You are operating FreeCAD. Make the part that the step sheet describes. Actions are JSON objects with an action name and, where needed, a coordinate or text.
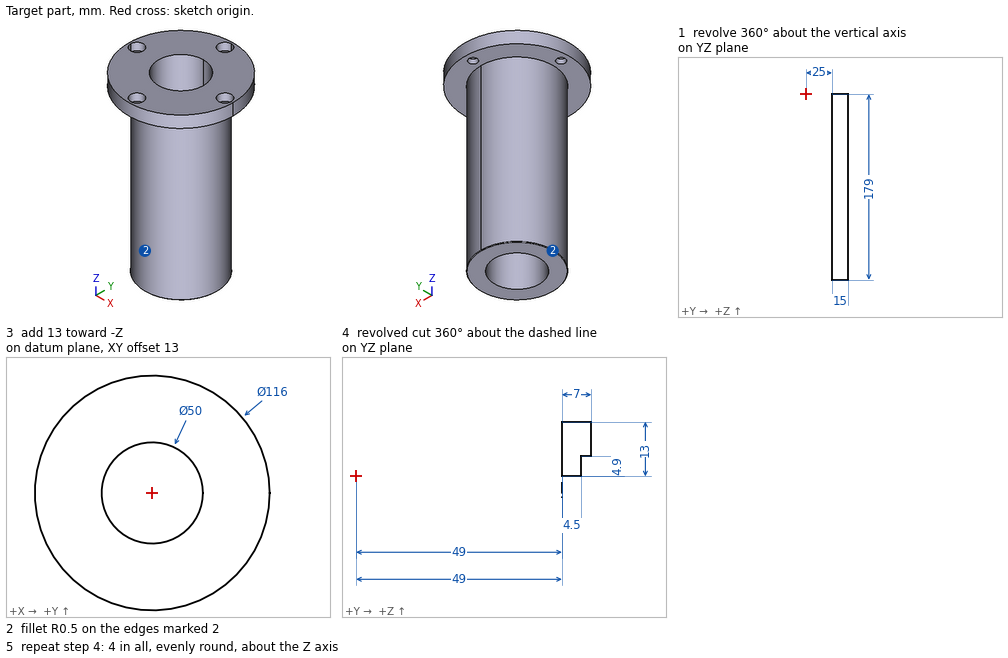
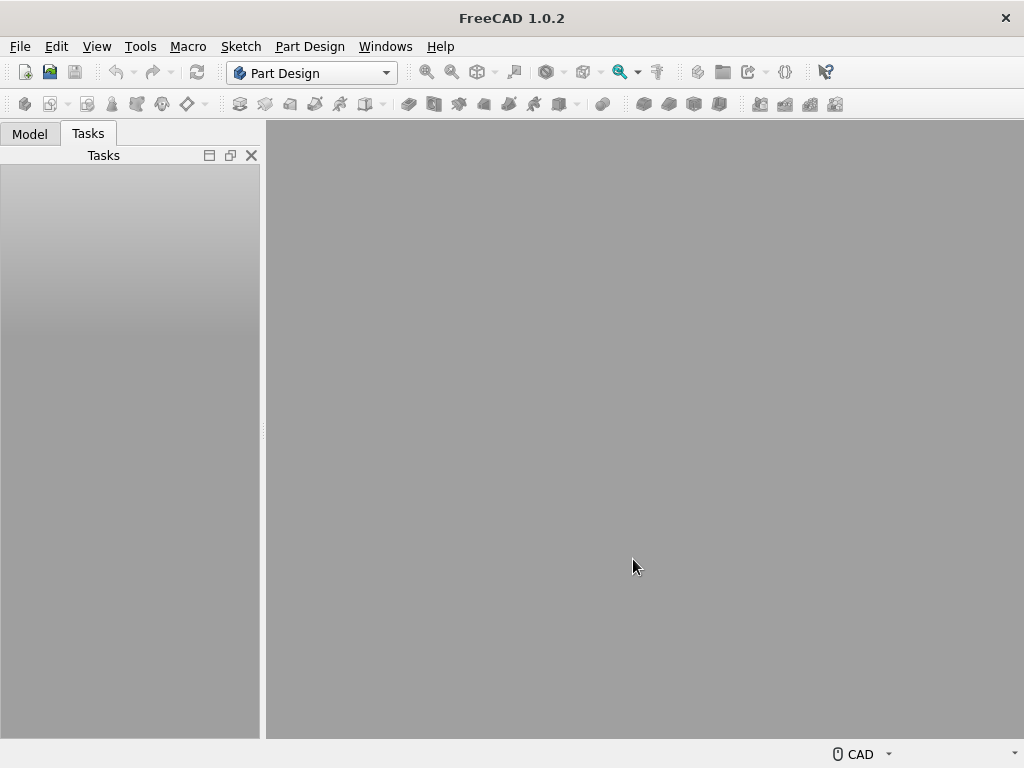
{"action": "left_click", "coordinate": [25, 72]}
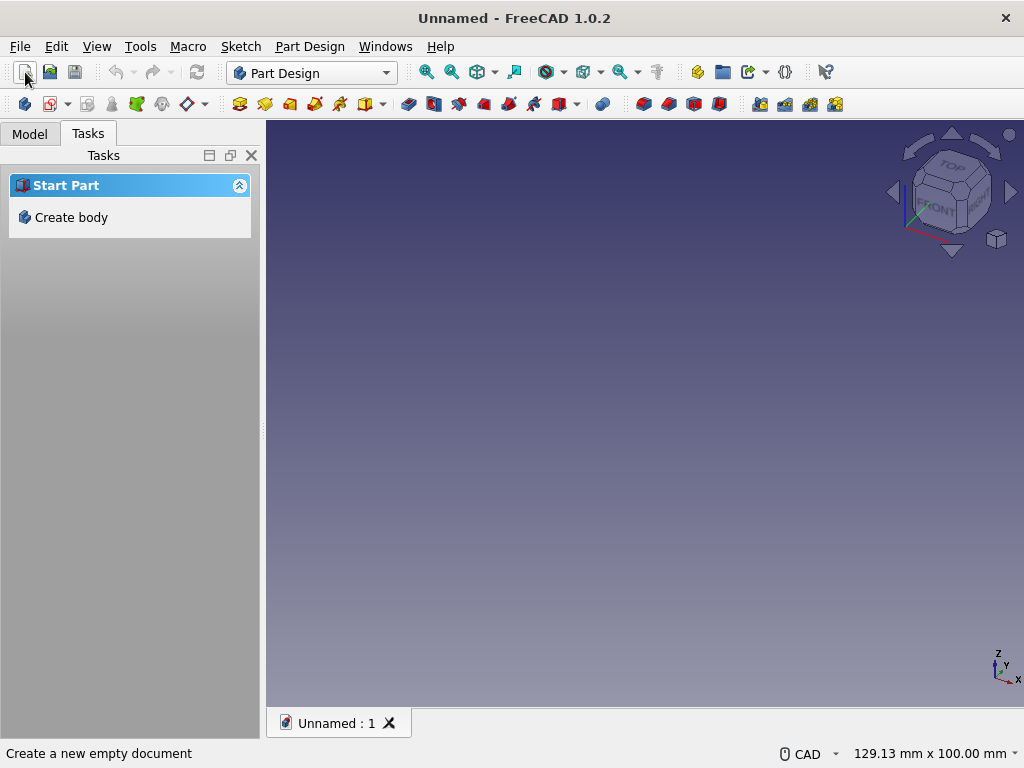
{"action": "left_click", "coordinate": [50, 104]}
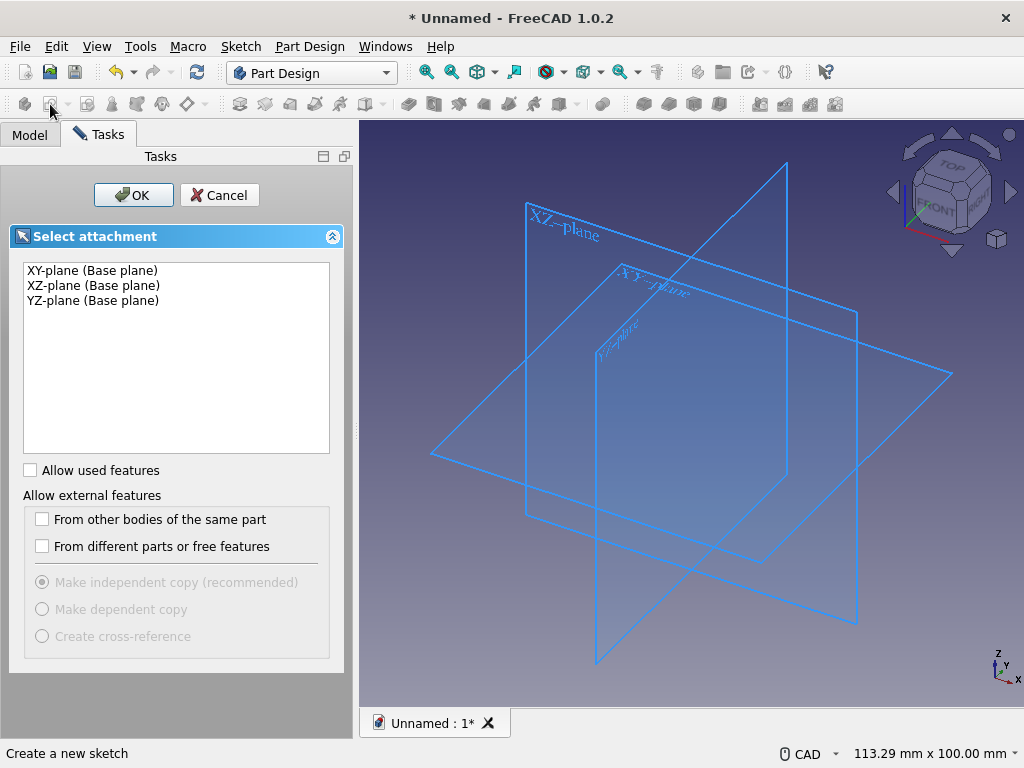
{"action": "left_click", "coordinate": [84, 300]}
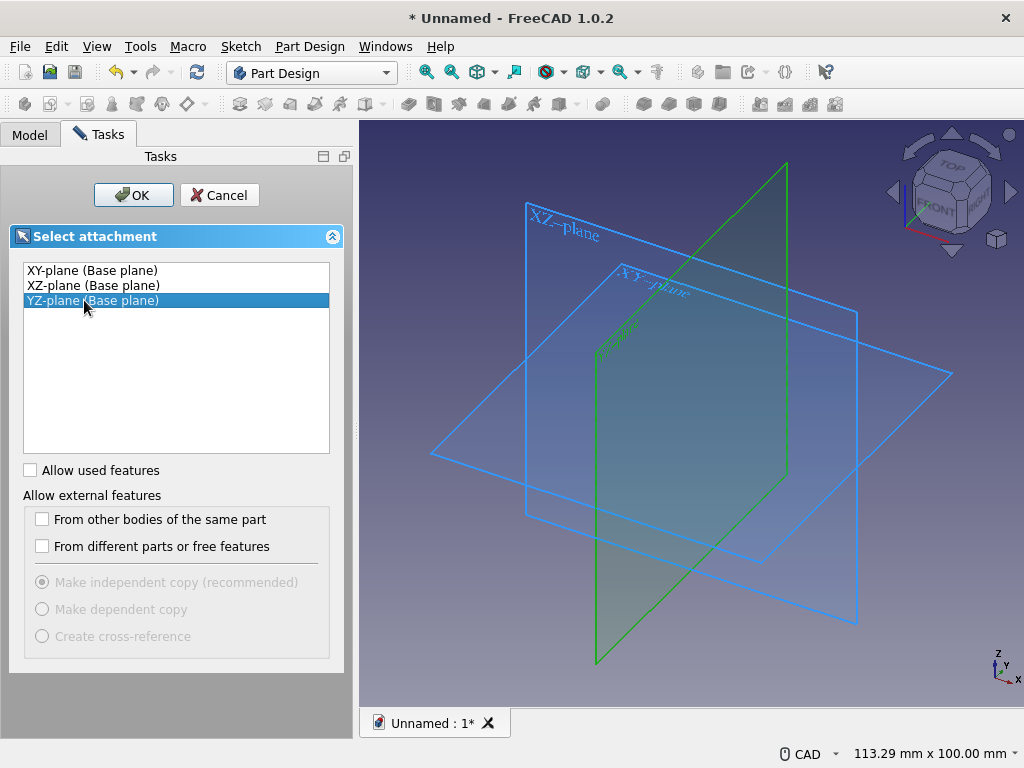
{"action": "left_click", "coordinate": [134, 195]}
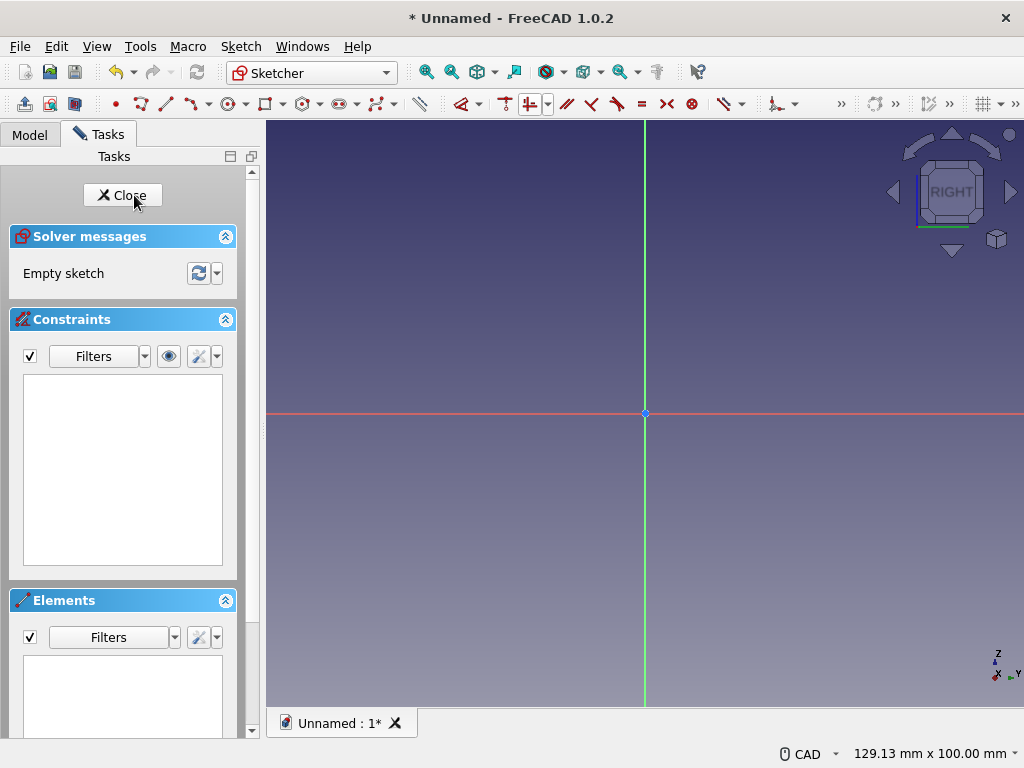
{"action": "scroll", "coordinate": [468, 148], "scroll_direction": "down", "scroll_amount": 5}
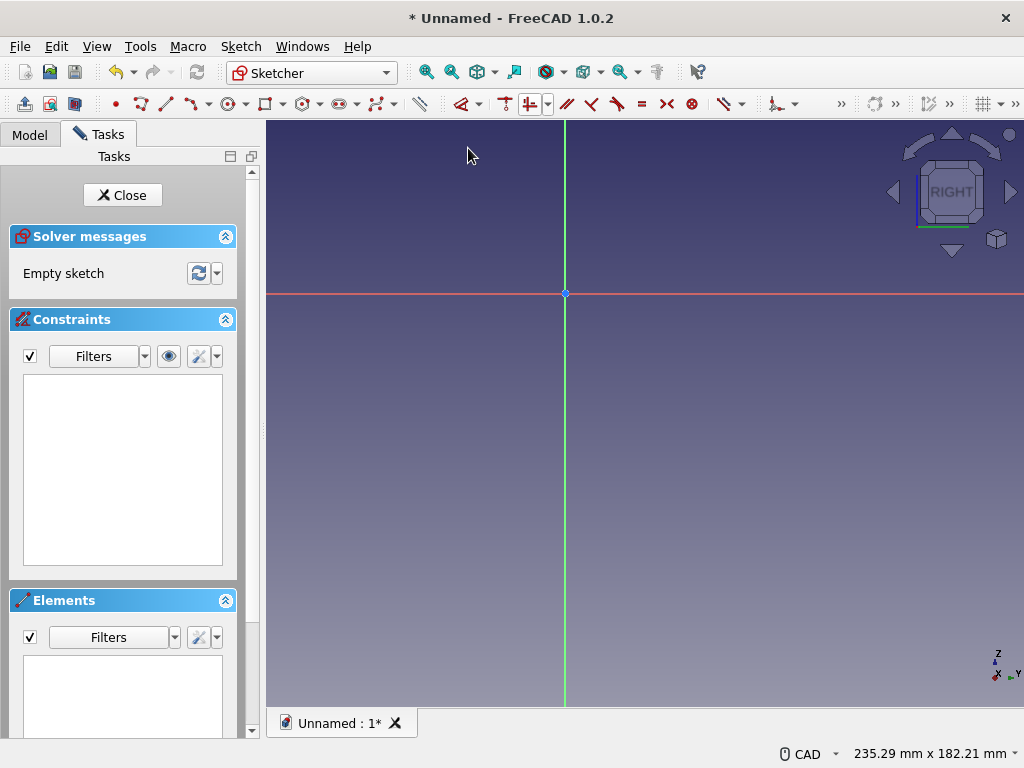
{"action": "left_click", "coordinate": [264, 104]}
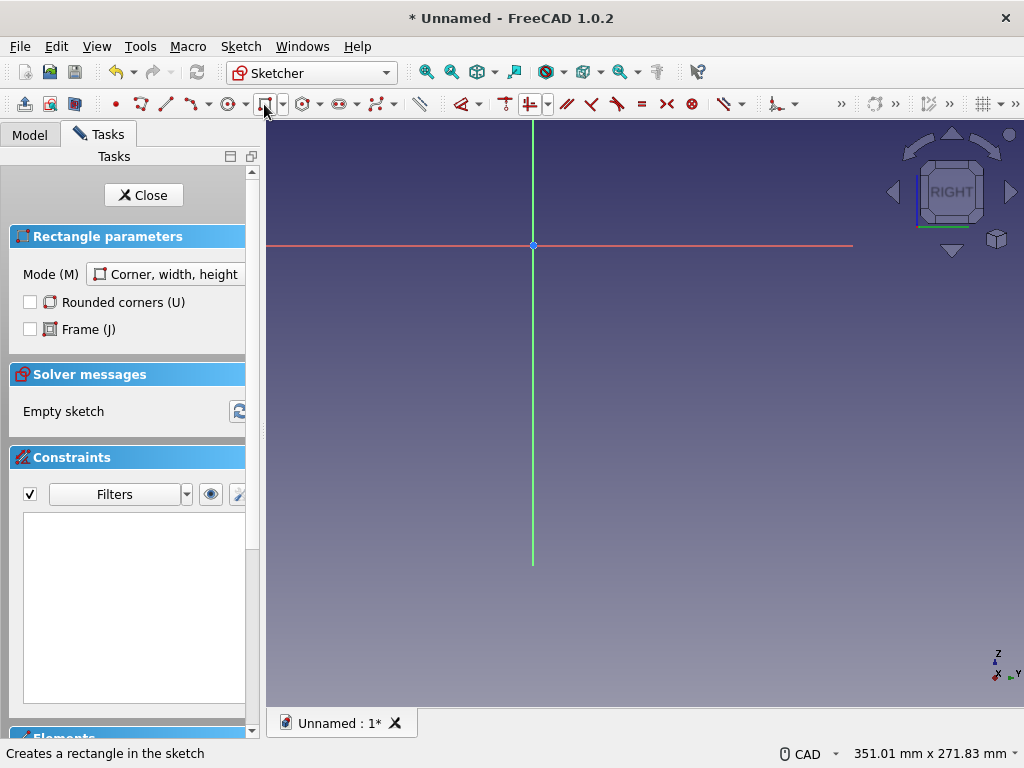
{"action": "left_click", "coordinate": [587, 246]}
{"action": "left_click", "coordinate": [620, 632]}
{"action": "key", "text": "Escape"}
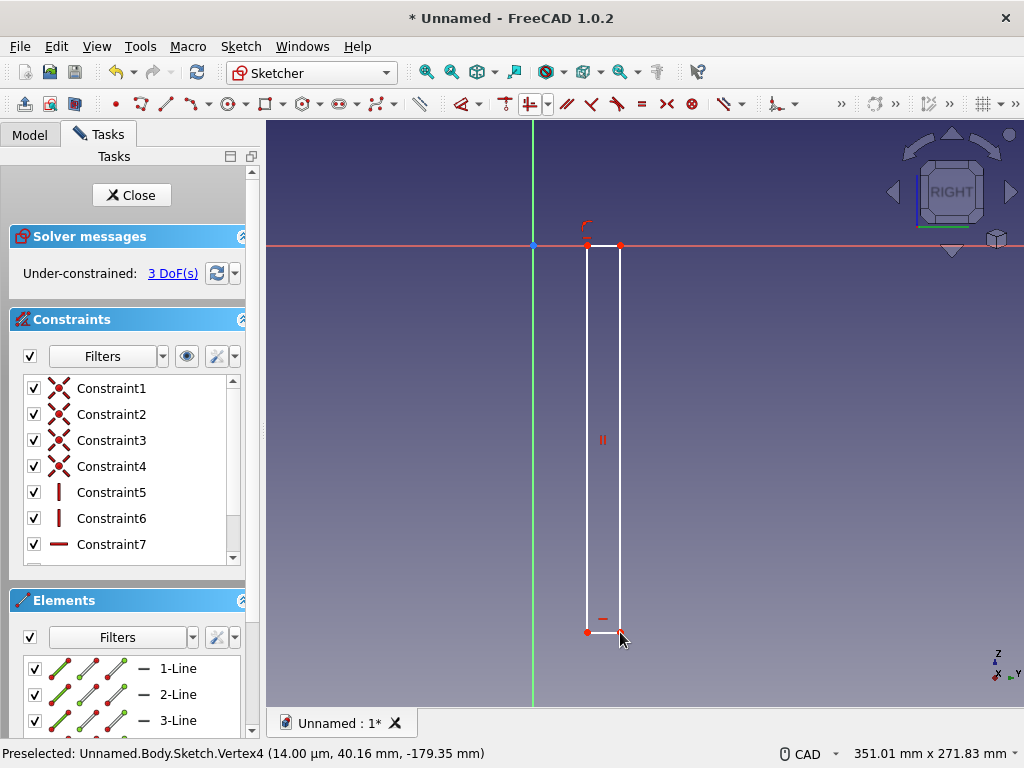
{"action": "left_click", "coordinate": [460, 104]}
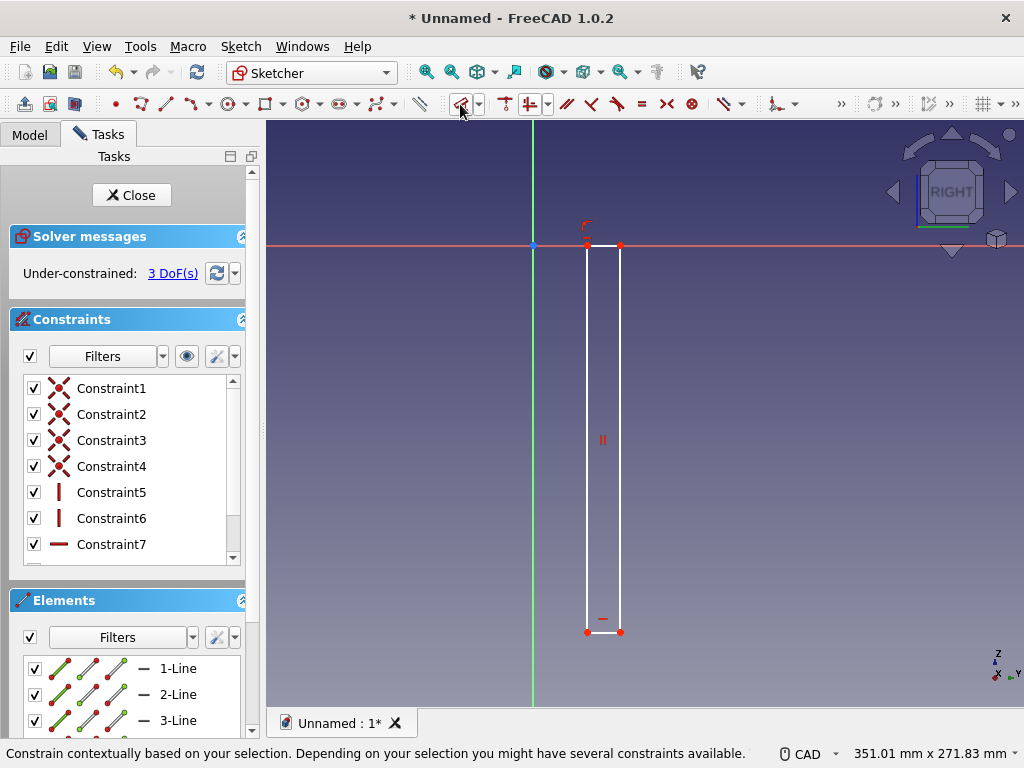
{"action": "scroll", "coordinate": [597, 633], "scroll_direction": "up", "scroll_amount": 2}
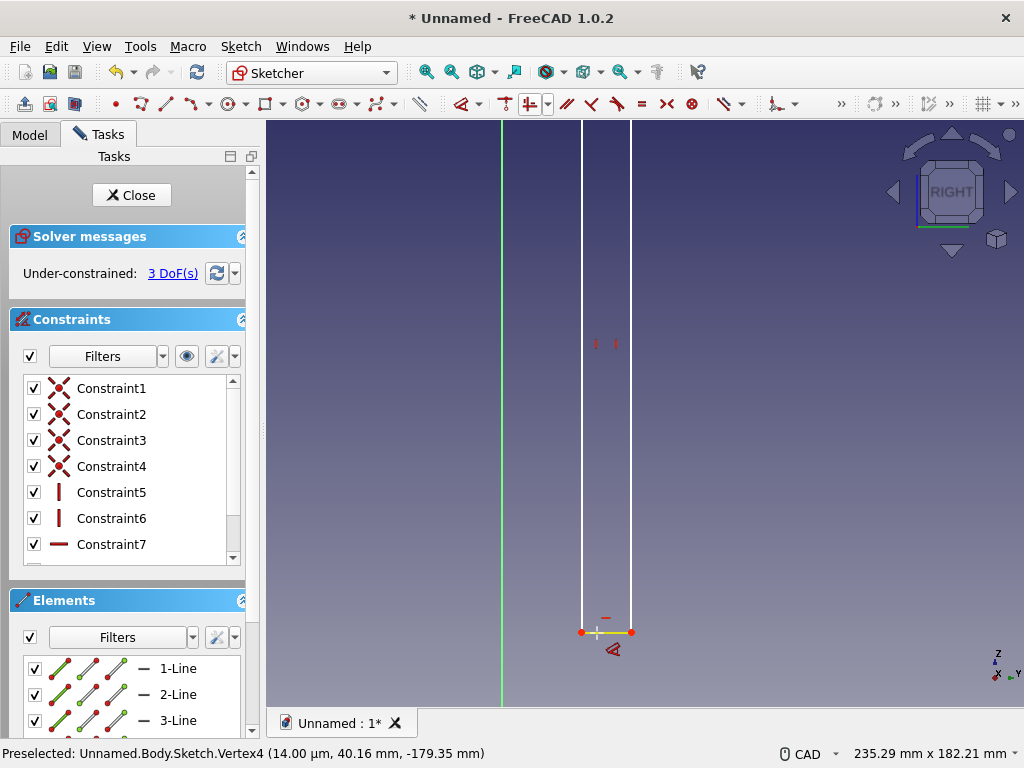
{"action": "left_click", "coordinate": [597, 633]}
{"action": "left_click", "coordinate": [606, 667]}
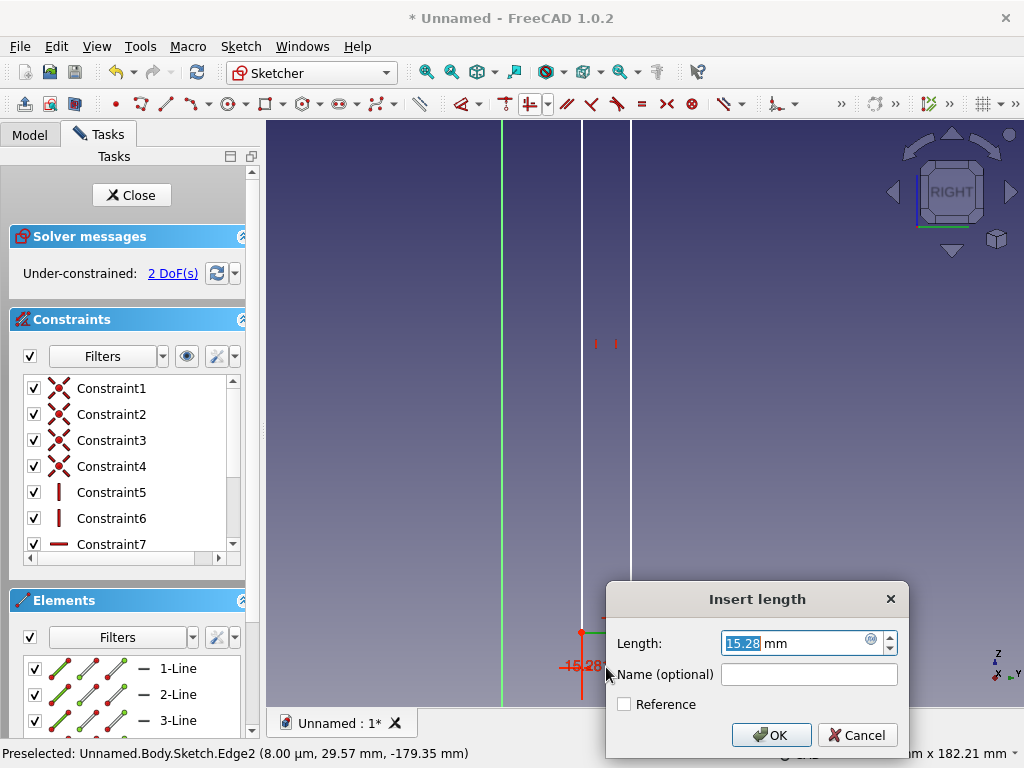
{"action": "type", "text": "15"}
{"action": "key", "text": "Return"}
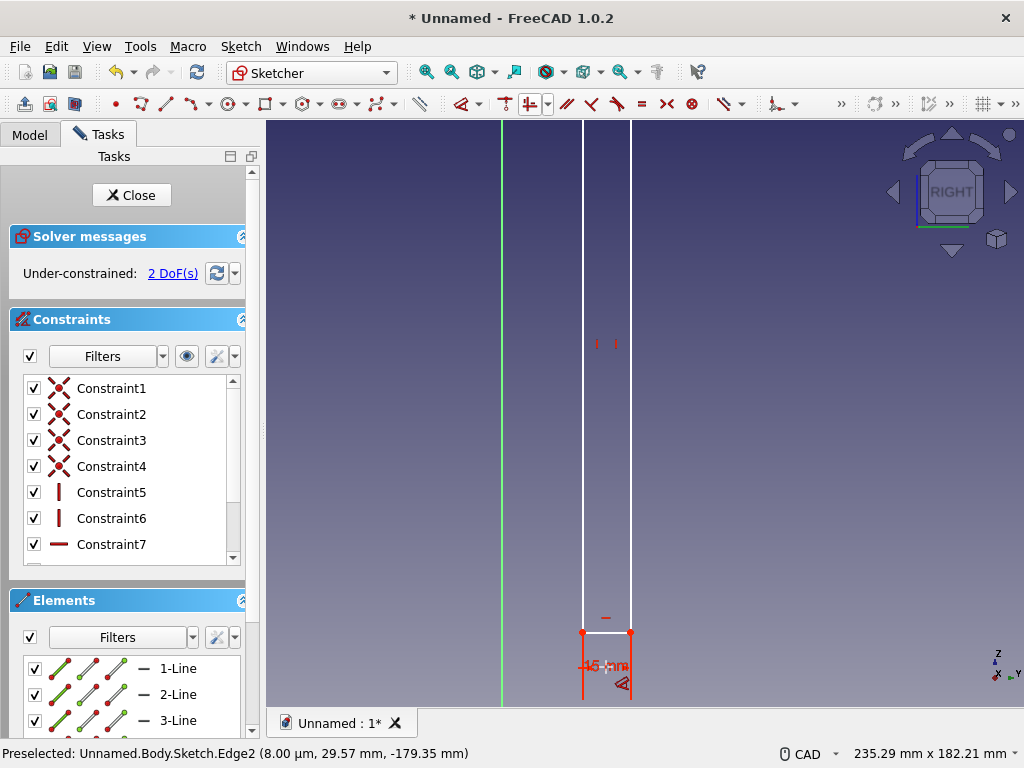
{"action": "left_click", "coordinate": [583, 228]}
{"action": "left_click", "coordinate": [617, 390]}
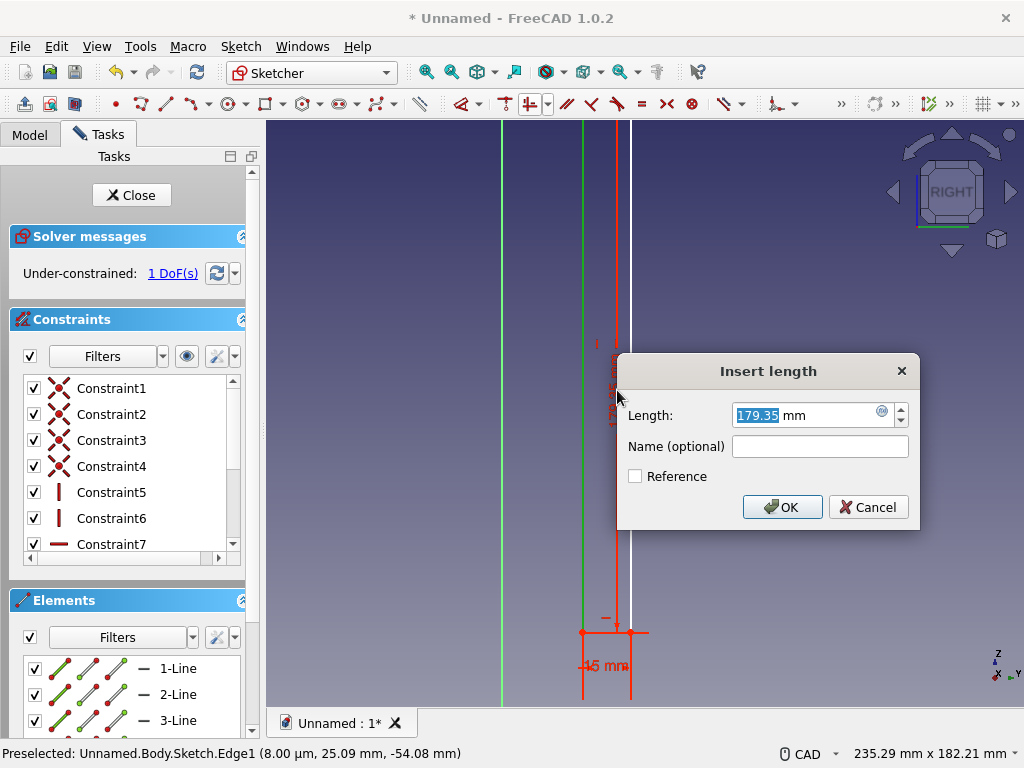
{"action": "type", "text": "179"}
{"action": "key", "text": "Return"}